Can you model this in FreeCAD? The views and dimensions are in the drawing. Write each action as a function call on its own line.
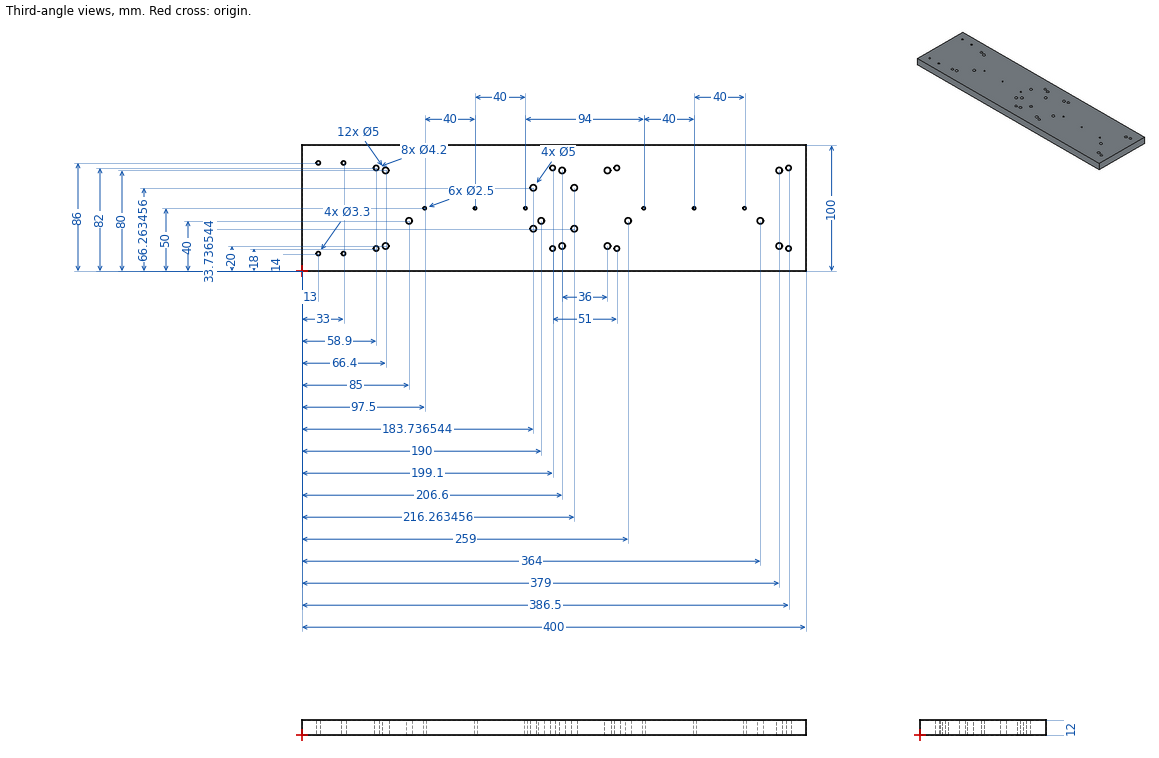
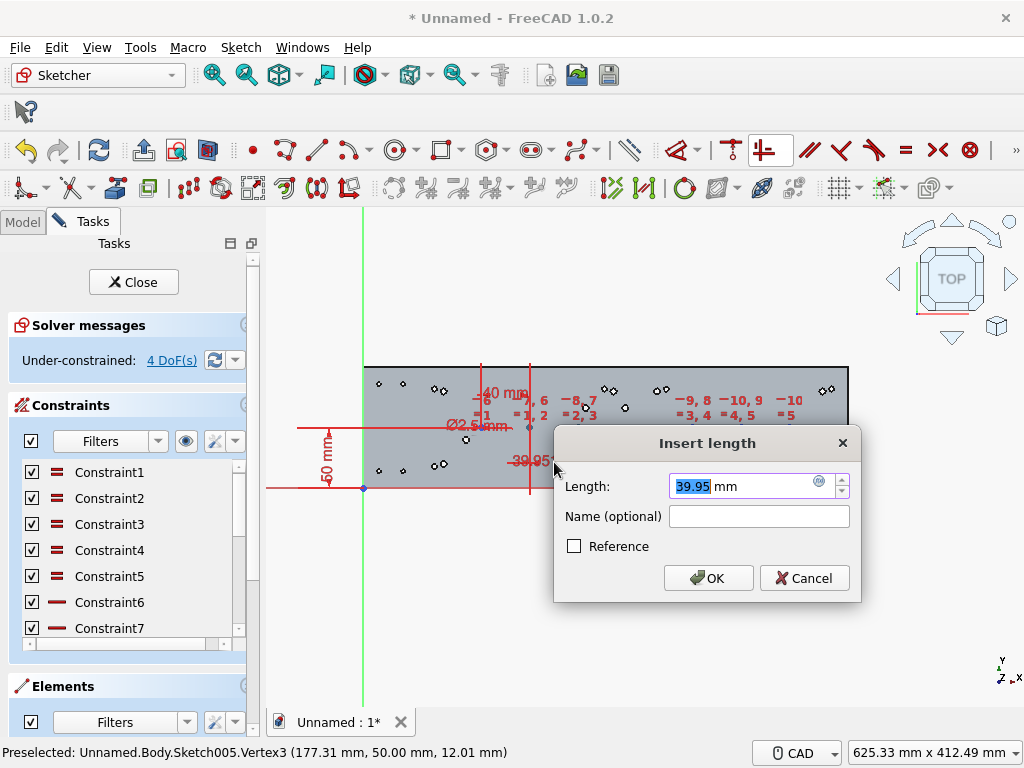
text(40)
key(Return)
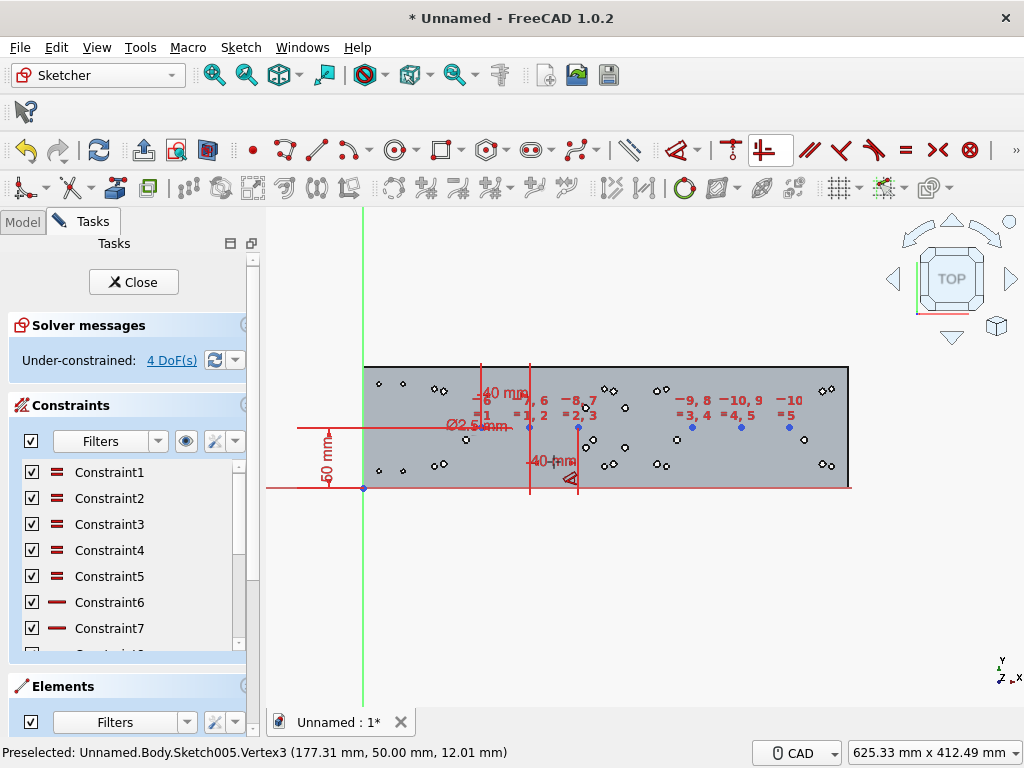
click(578, 428)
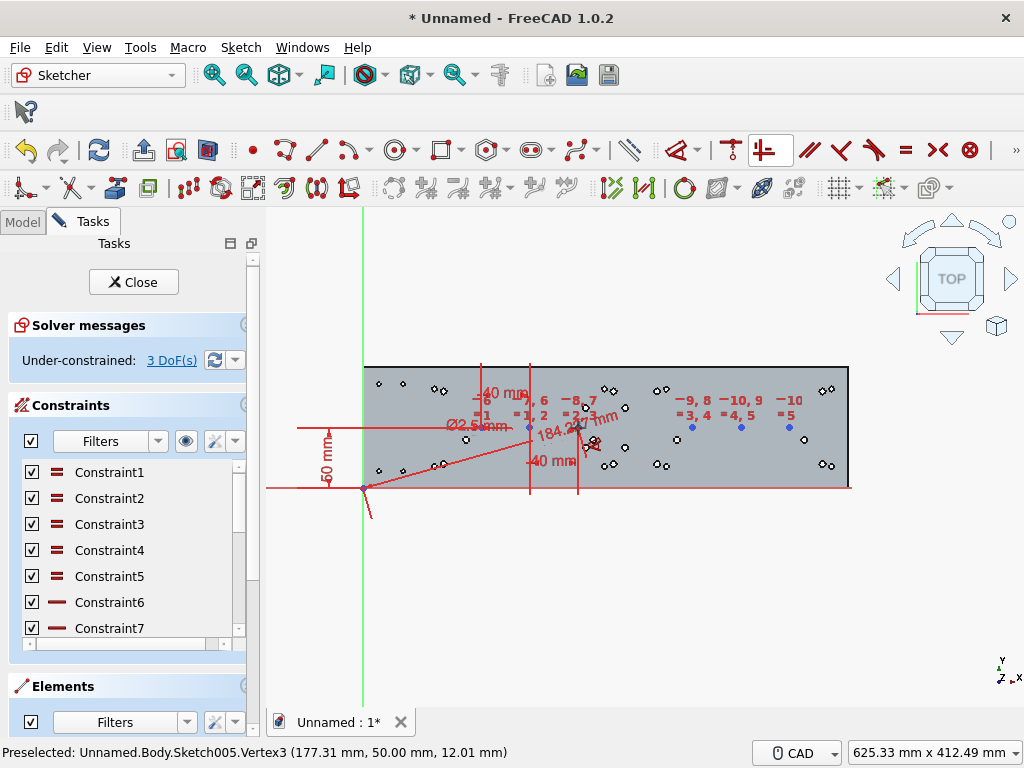
click(692, 428)
click(635, 394)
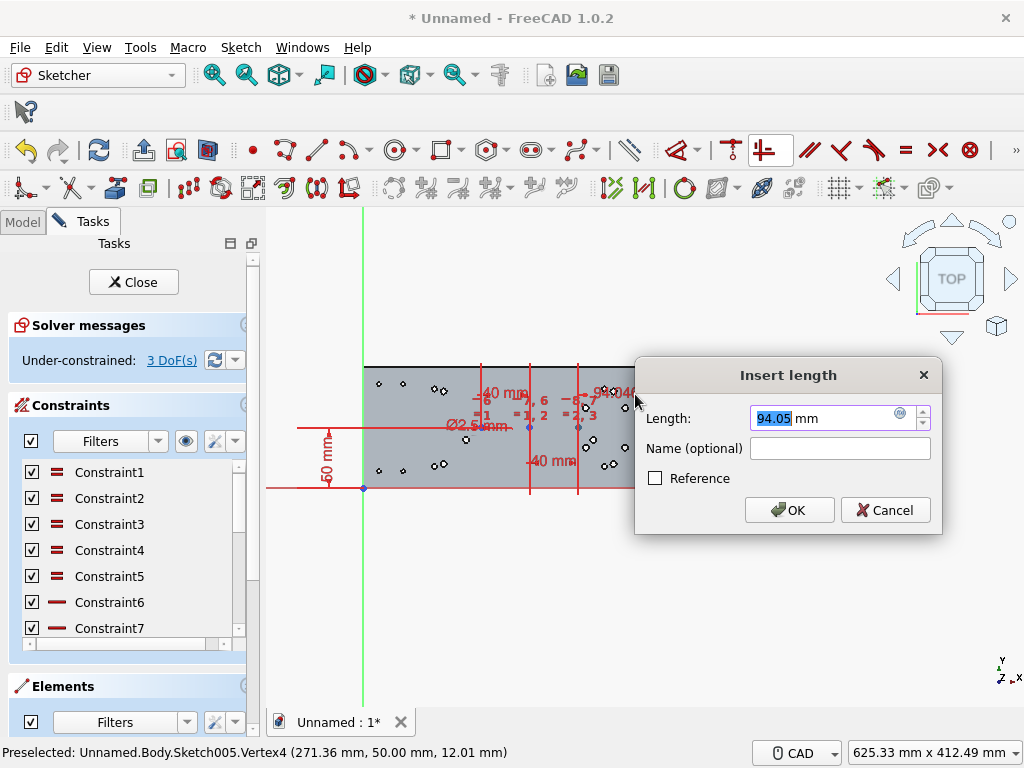
text(94)
key(Return)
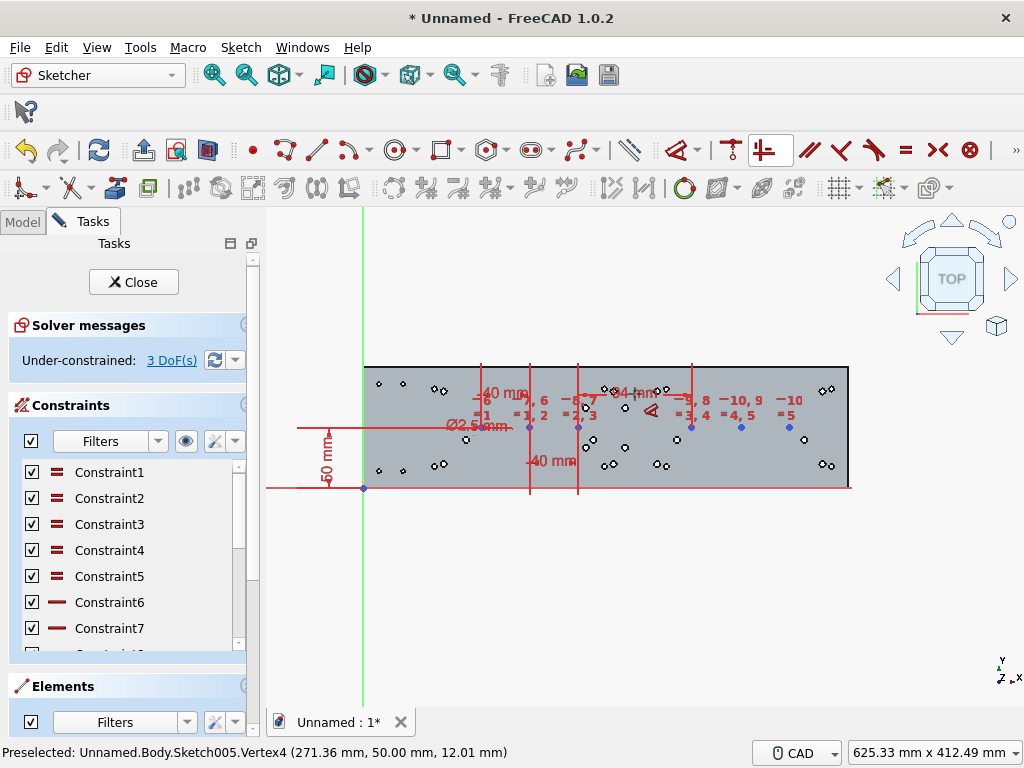
click(692, 428)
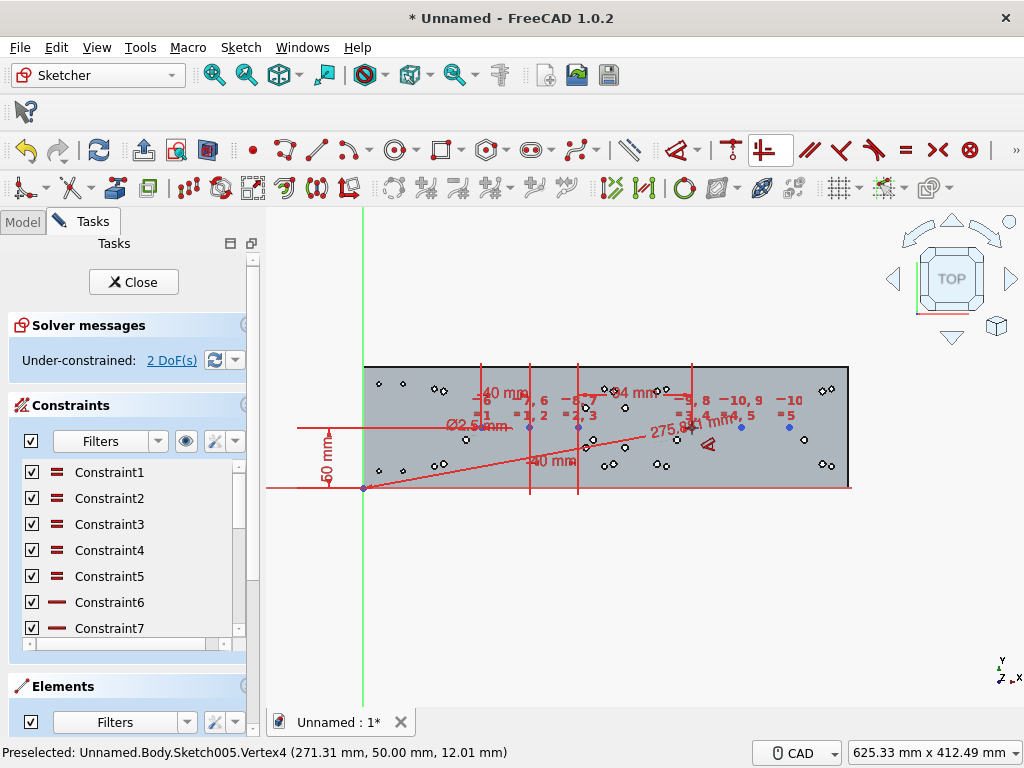
click(741, 428)
click(716, 394)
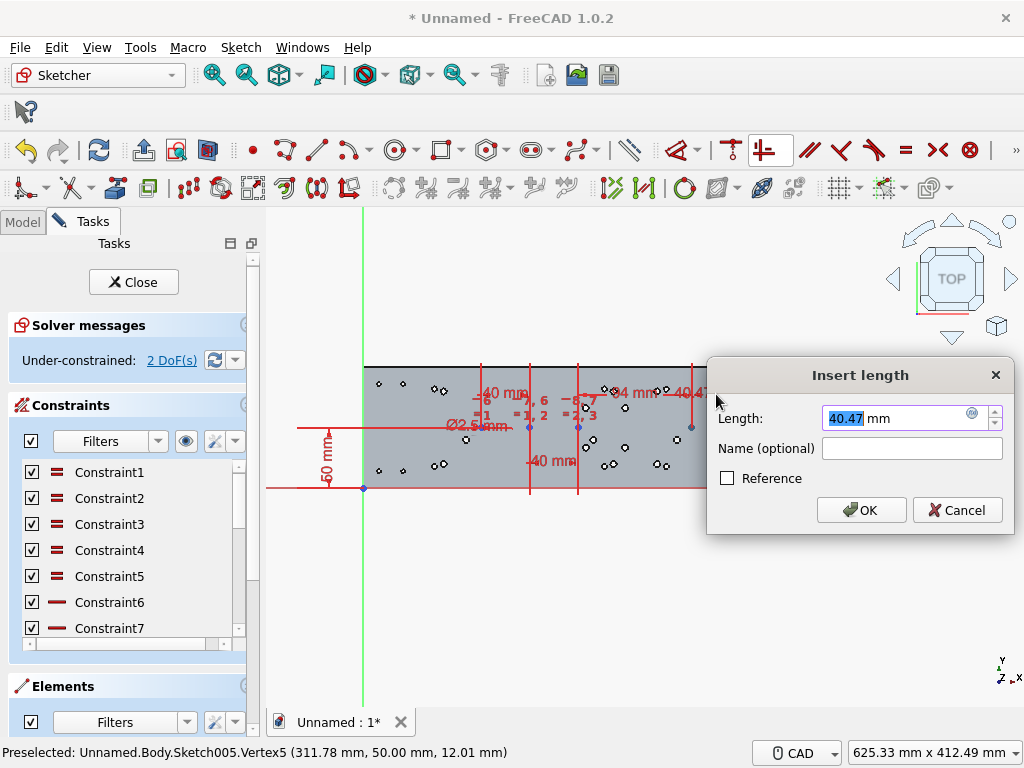
text(40)
key(Return)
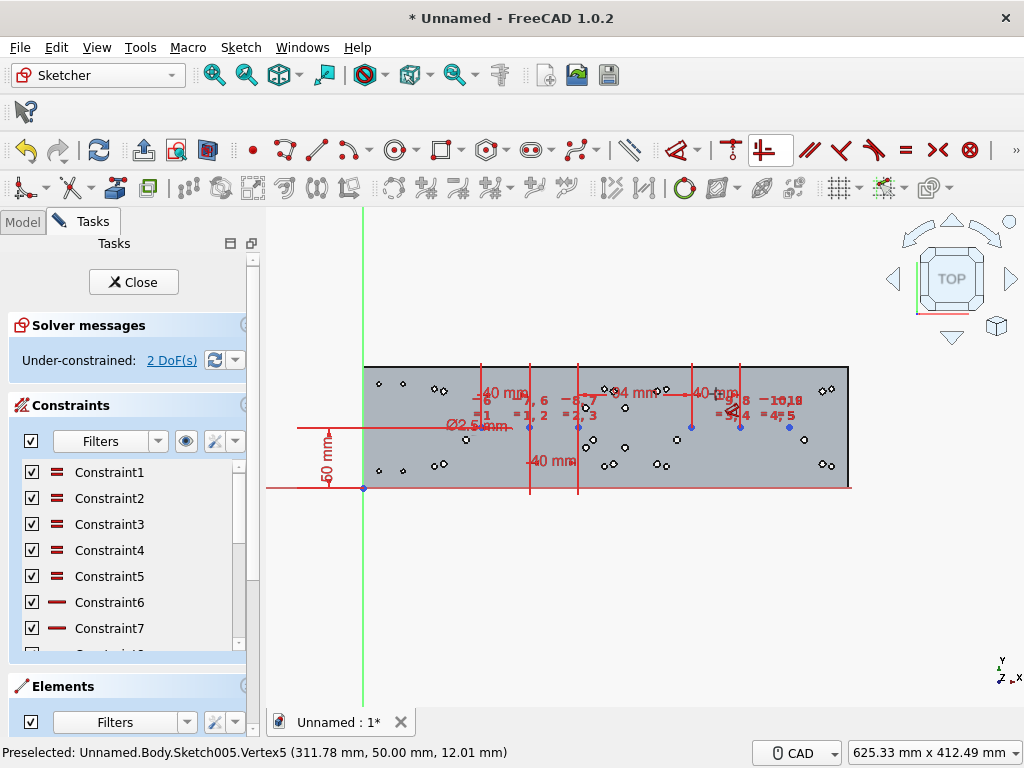
click(740, 428)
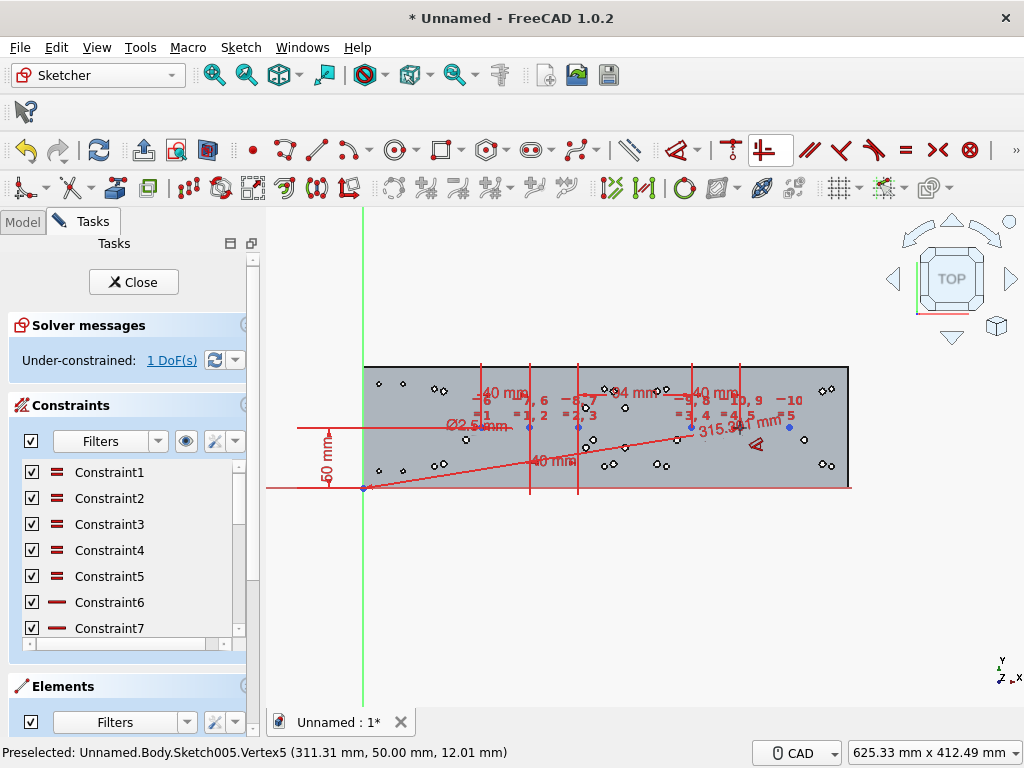
click(789, 428)
click(765, 462)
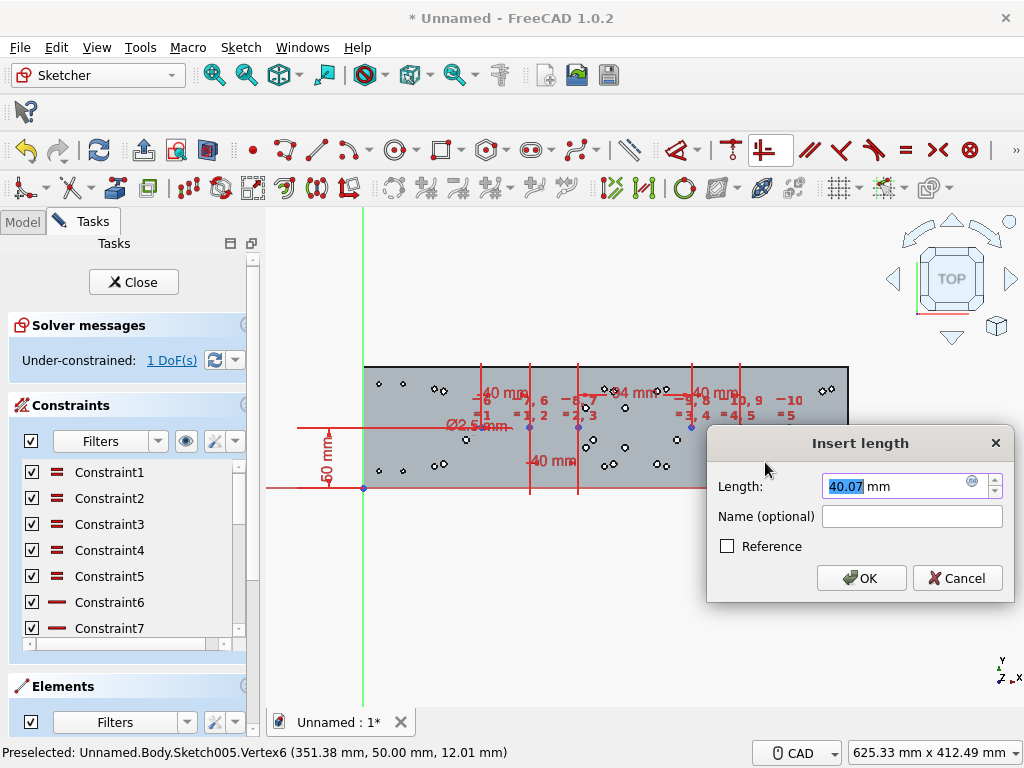
text(40)
key(Return)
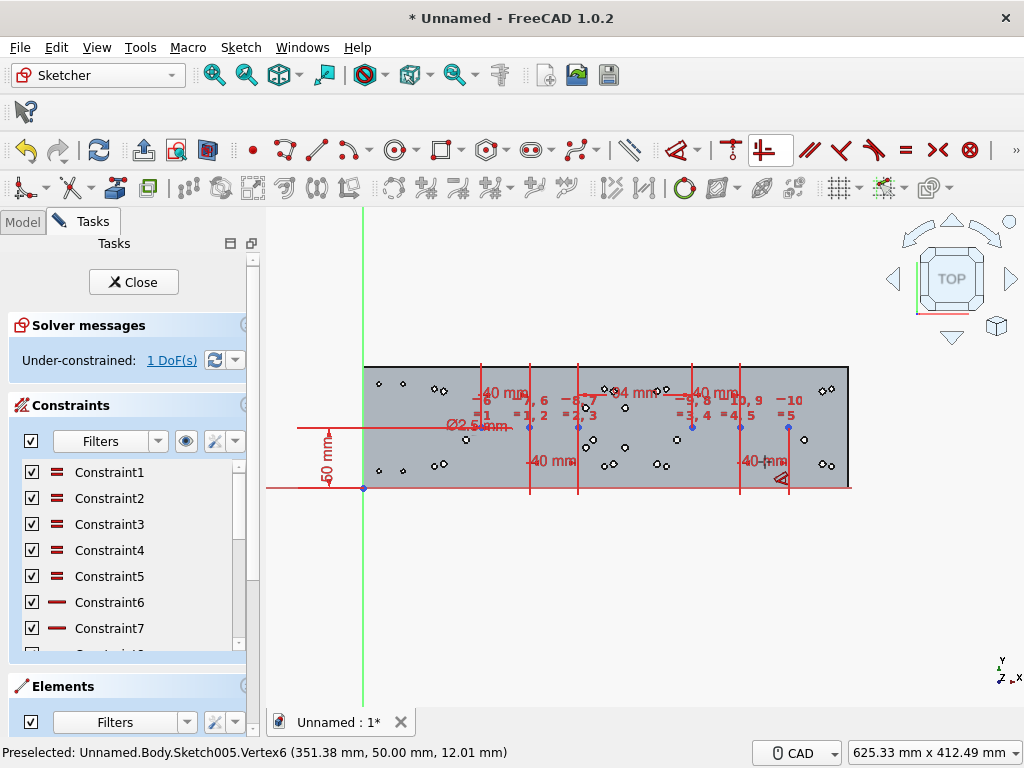
click(481, 428)
click(422, 522)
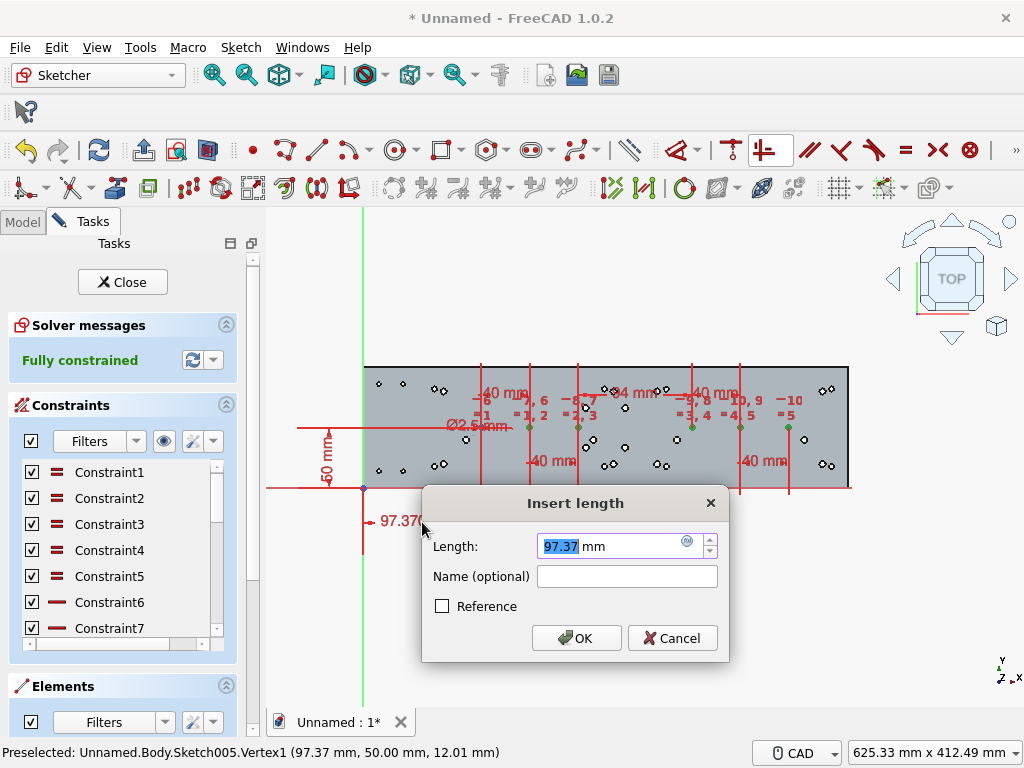
text(97.5)
key(Return)
key(Escape)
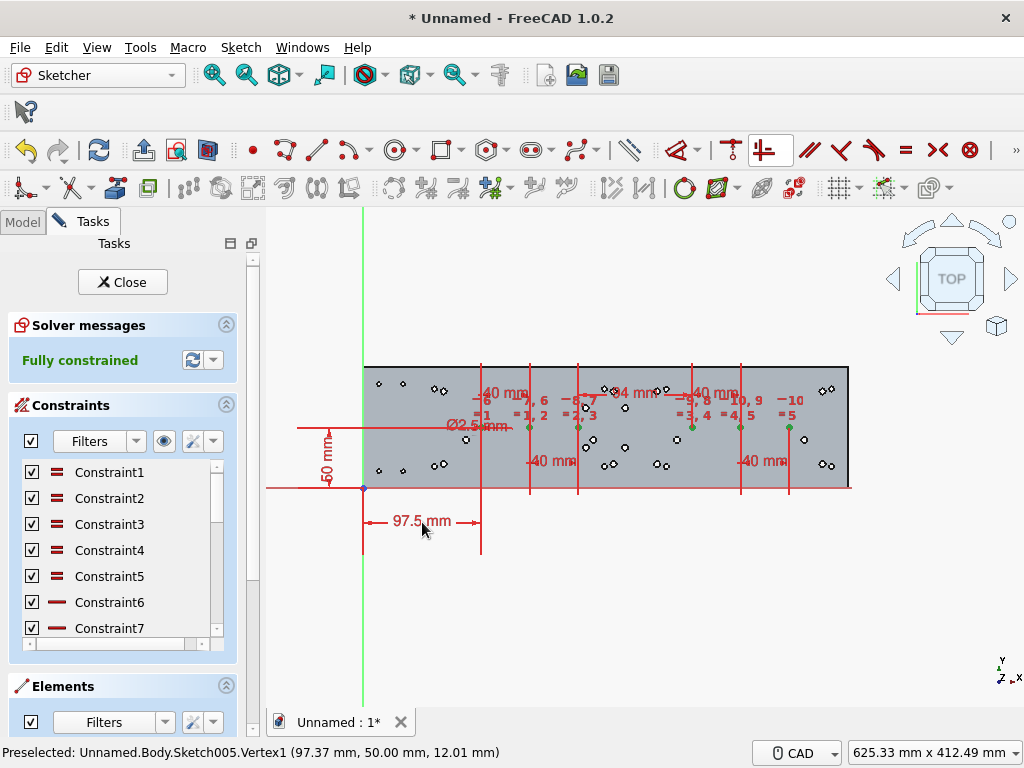
click(123, 282)